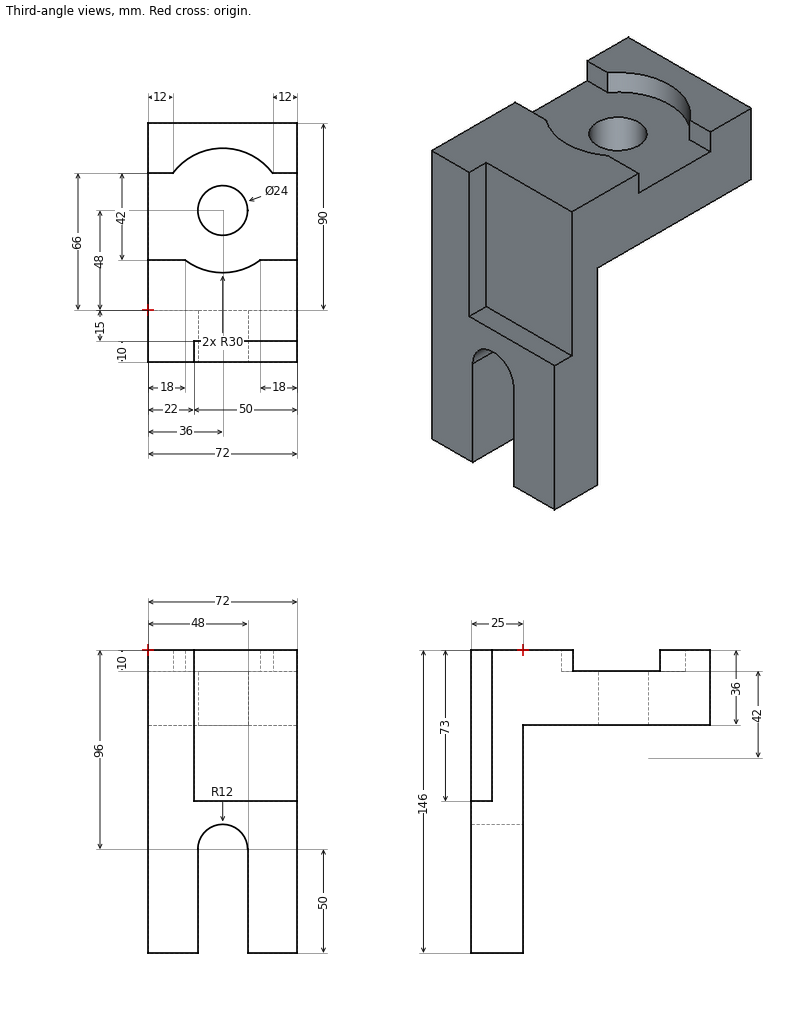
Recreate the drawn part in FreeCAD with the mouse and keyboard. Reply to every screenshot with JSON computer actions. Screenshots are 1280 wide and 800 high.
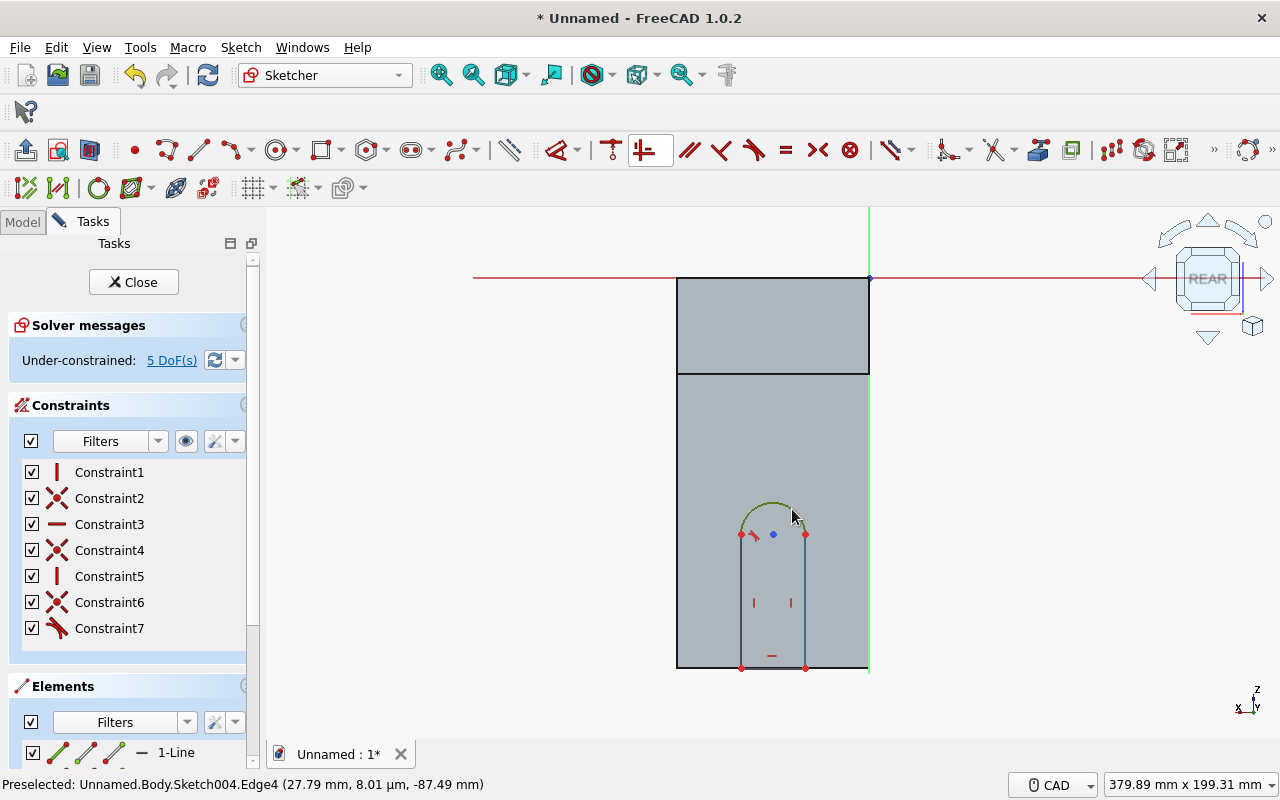
{"action": "left_click", "coordinate": [754, 150]}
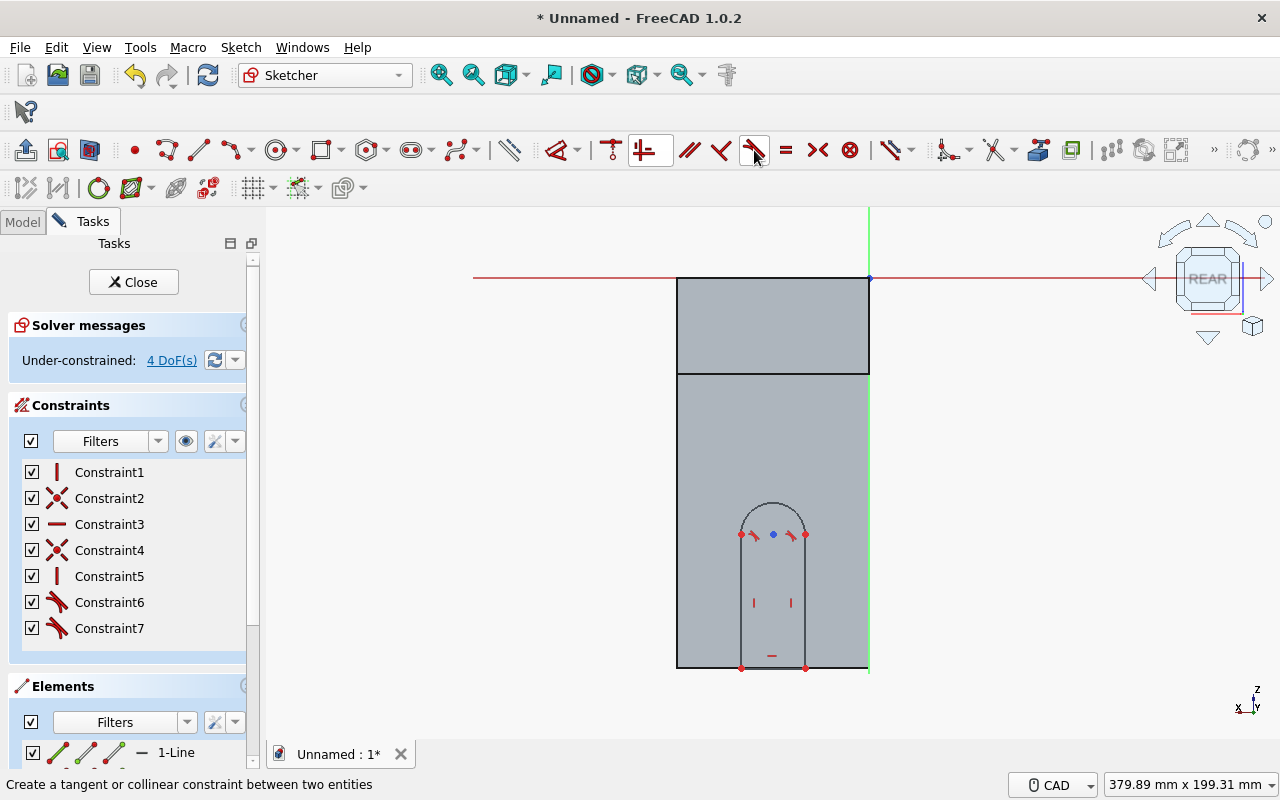
{"action": "left_click", "coordinate": [556, 150]}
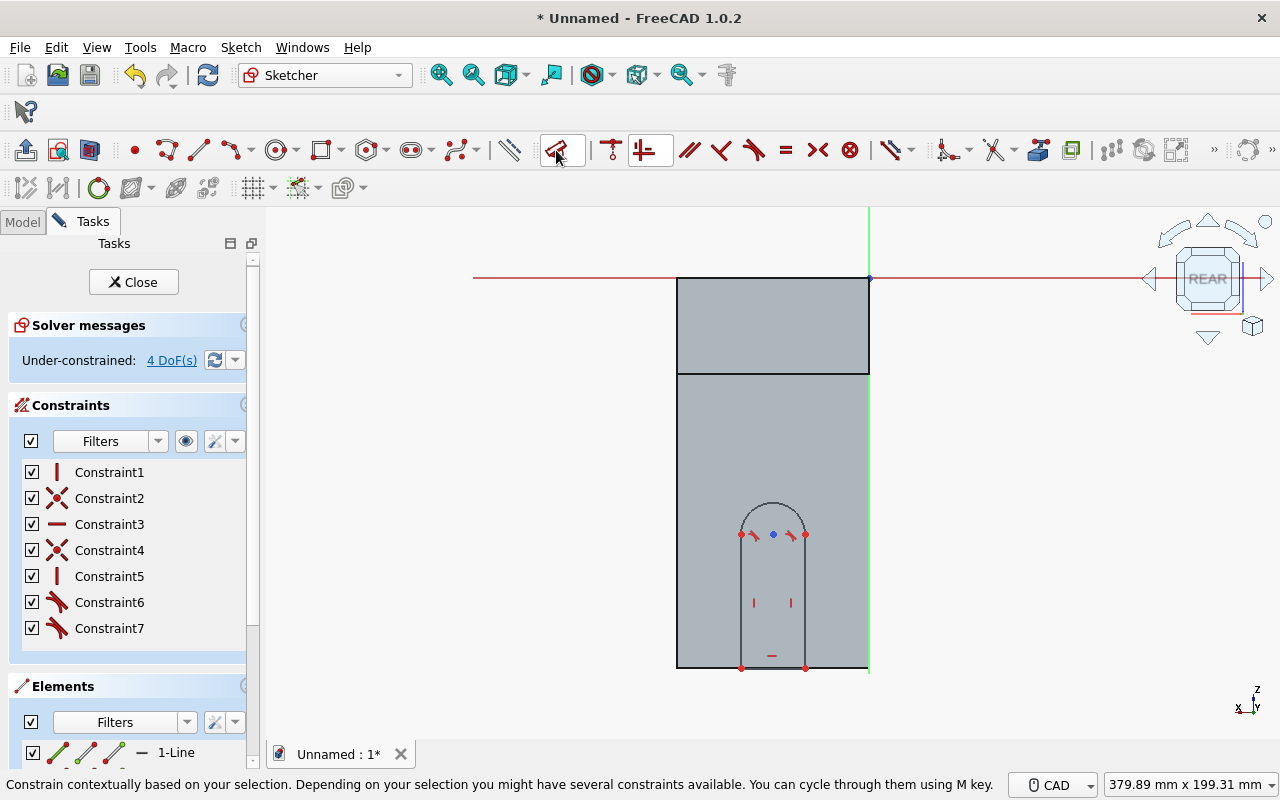
{"action": "scroll", "coordinate": [792, 509], "scroll_direction": "up", "scroll_amount": 2}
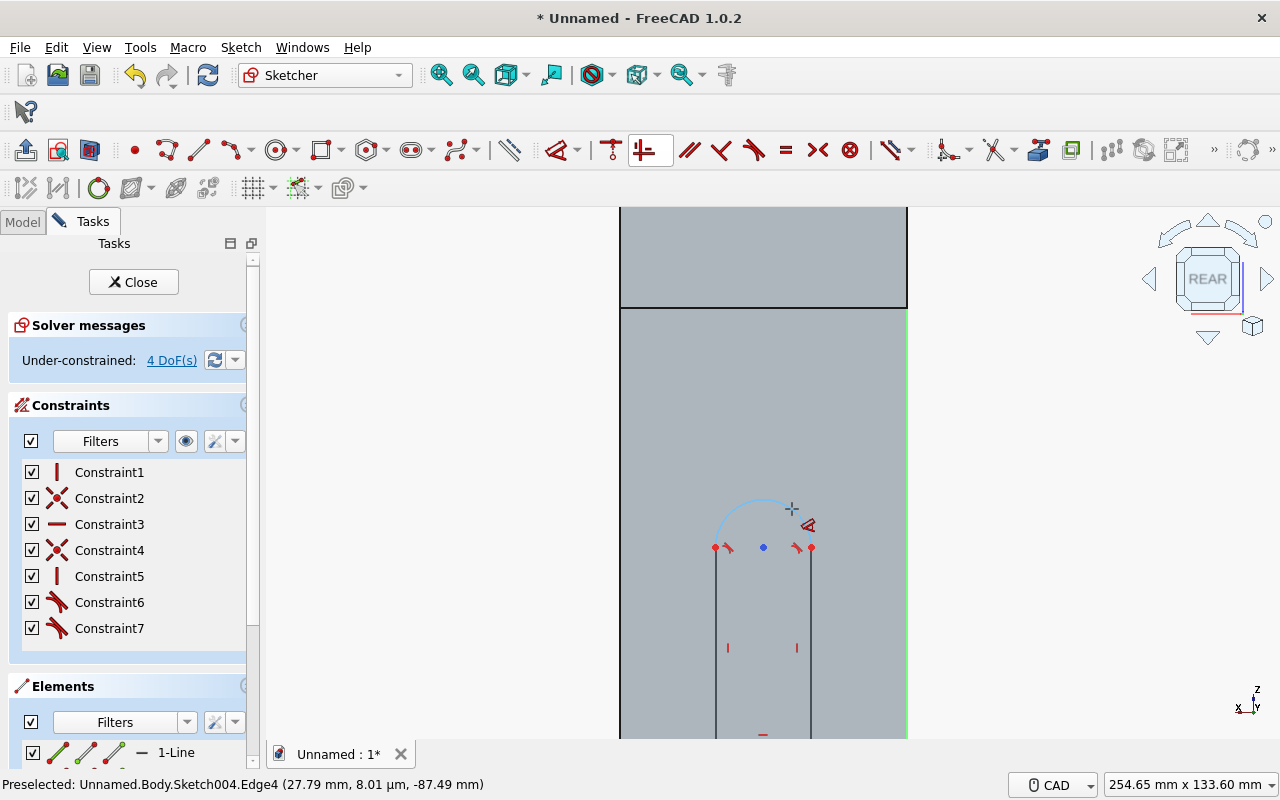
{"action": "left_click", "coordinate": [791, 509]}
{"action": "left_click", "coordinate": [810, 483]}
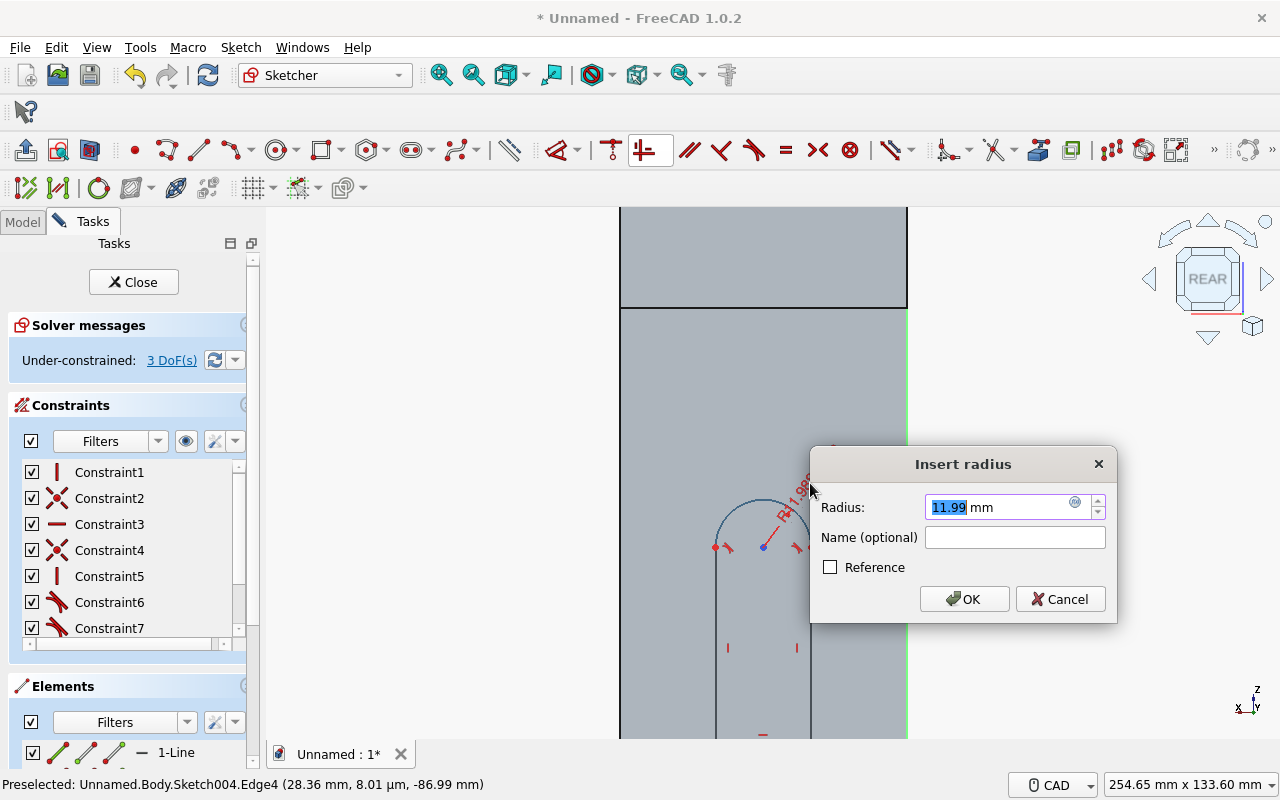
{"action": "type", "text": "12"}
{"action": "key", "text": "Return"}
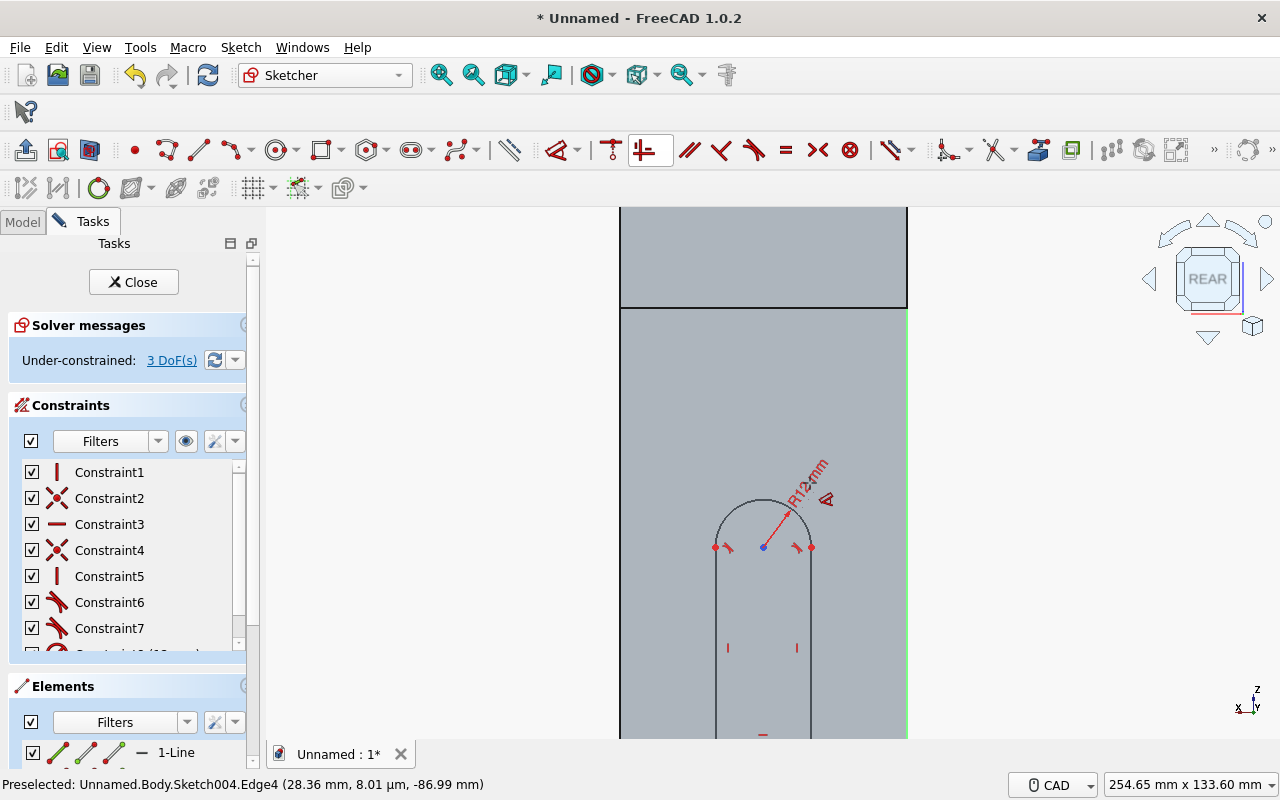
{"action": "left_click", "coordinate": [716, 607]}
{"action": "left_click", "coordinate": [682, 629]}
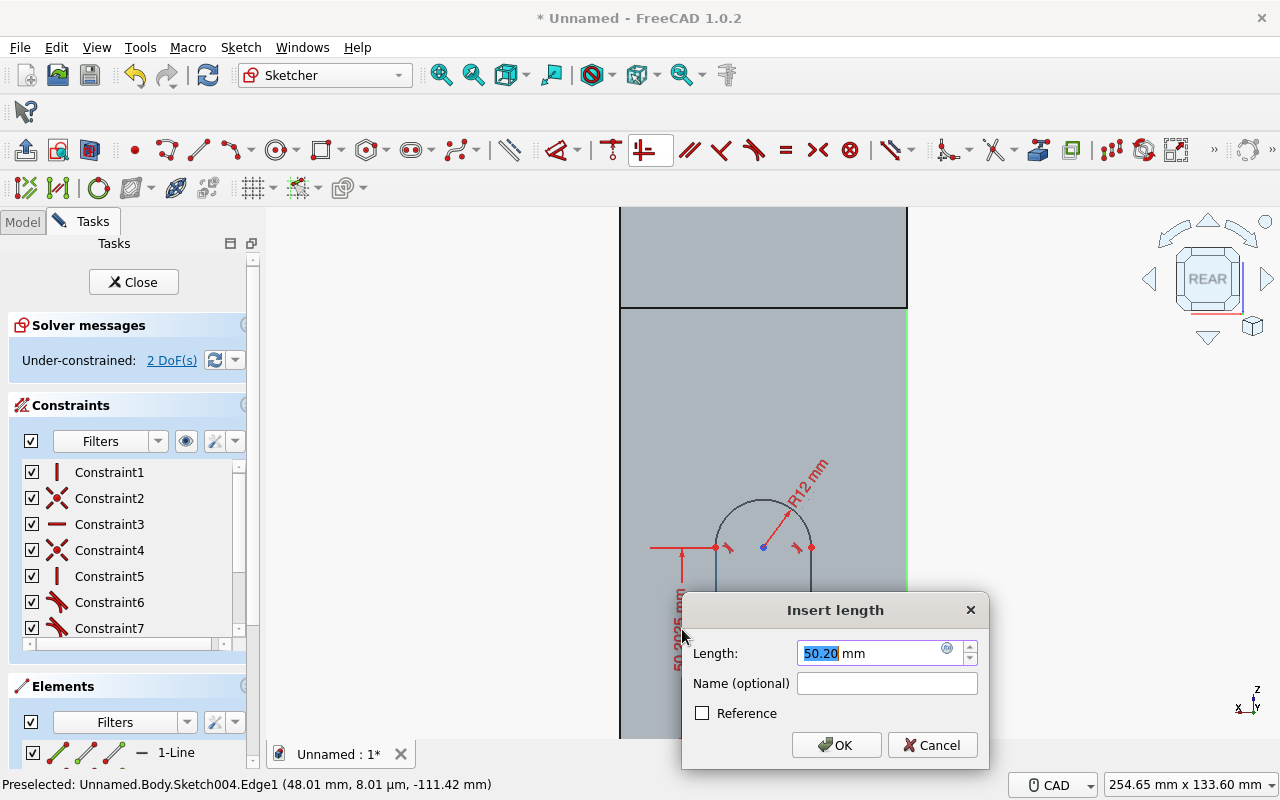
{"action": "type", "text": "50"}
{"action": "key", "text": "Return"}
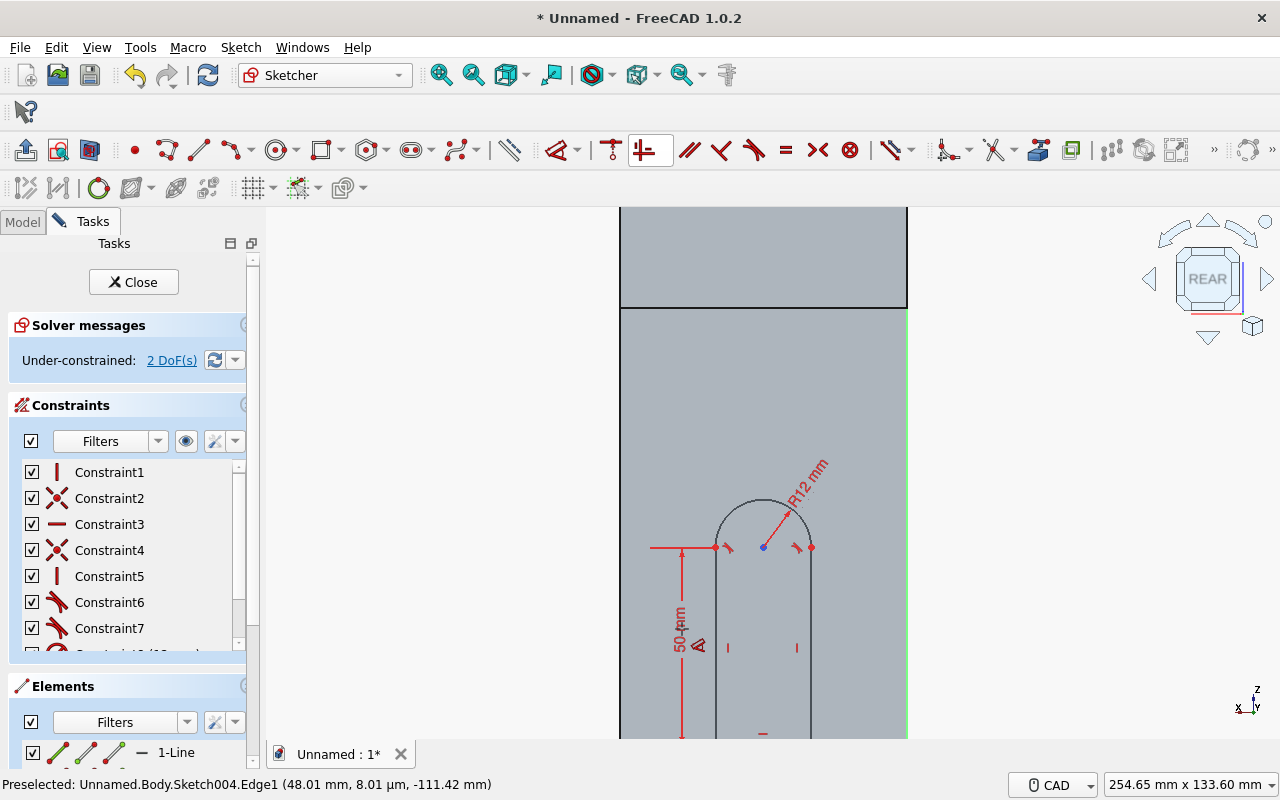
{"action": "left_click", "coordinate": [716, 548]}
{"action": "left_click", "coordinate": [767, 582]}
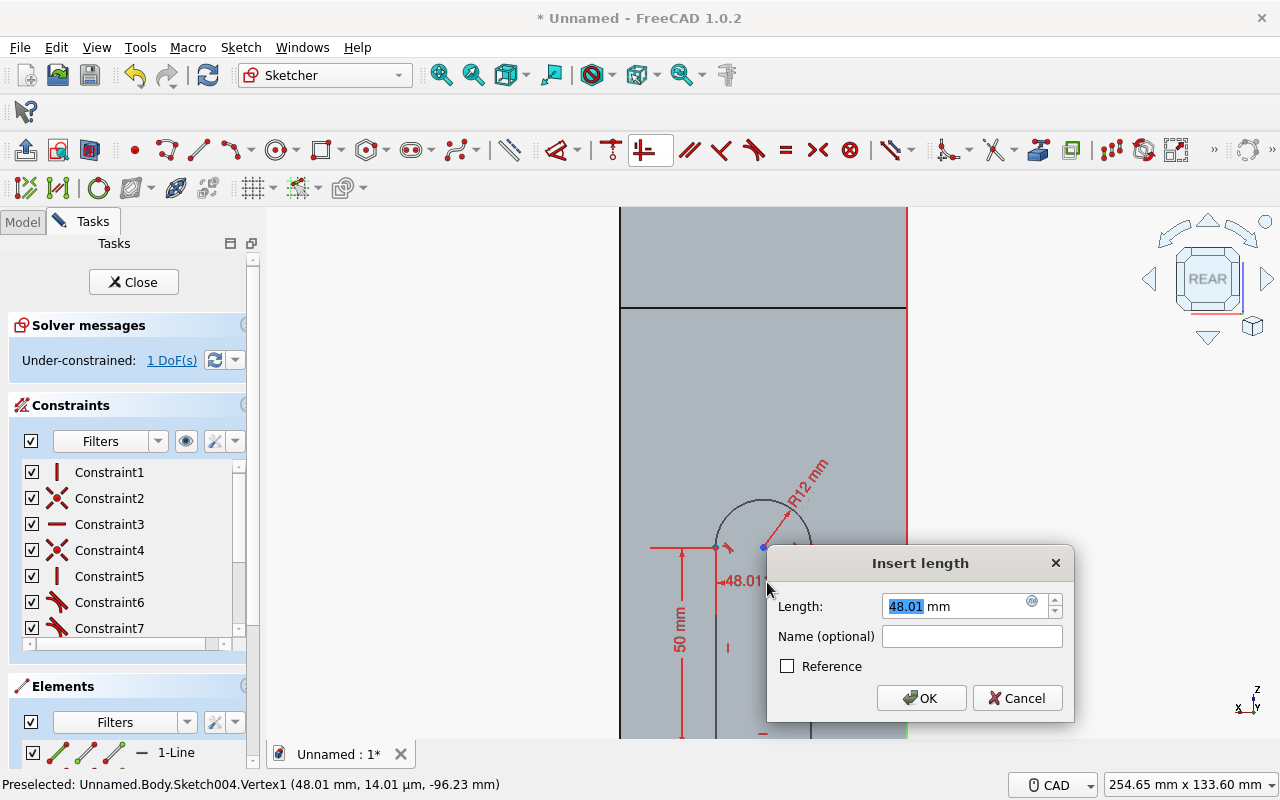
{"action": "type", "text": "48"}
{"action": "key", "text": "Return"}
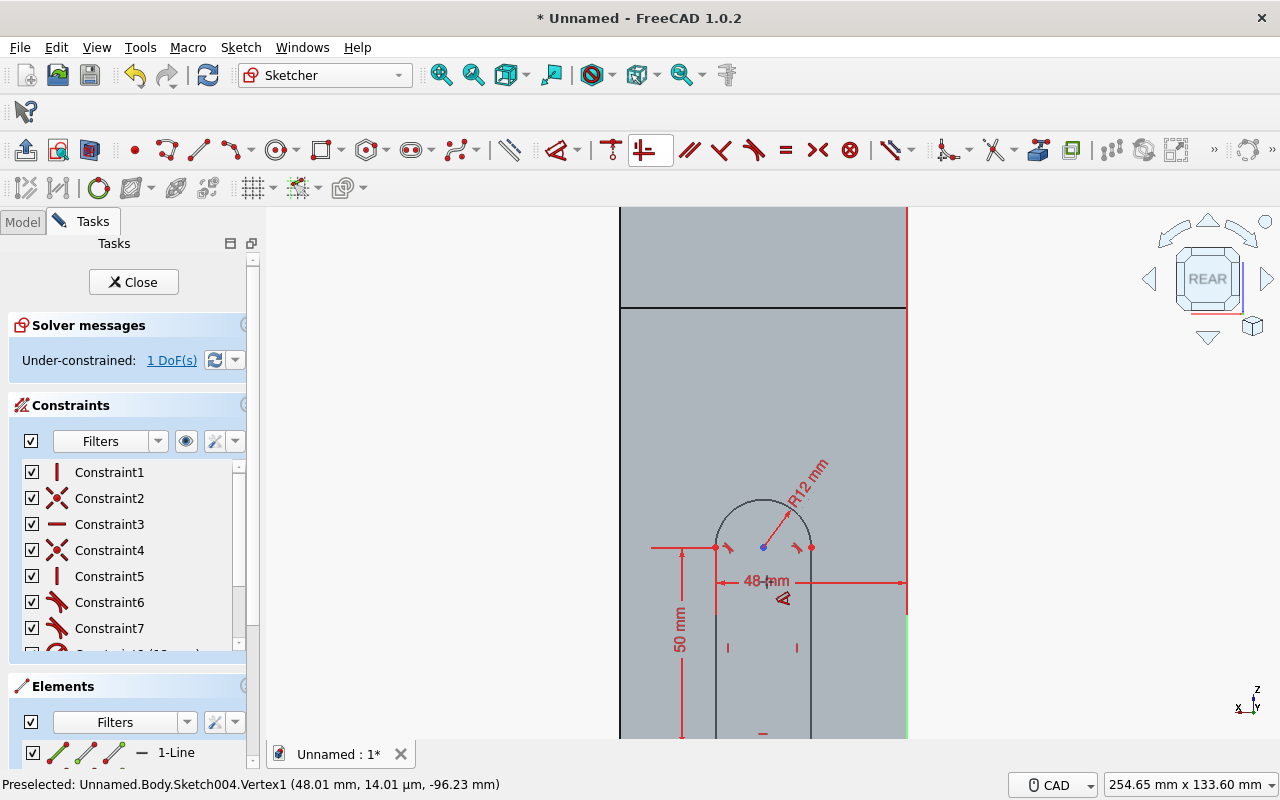
{"action": "left_click", "coordinate": [716, 548]}
{"action": "left_click", "coordinate": [941, 391]}